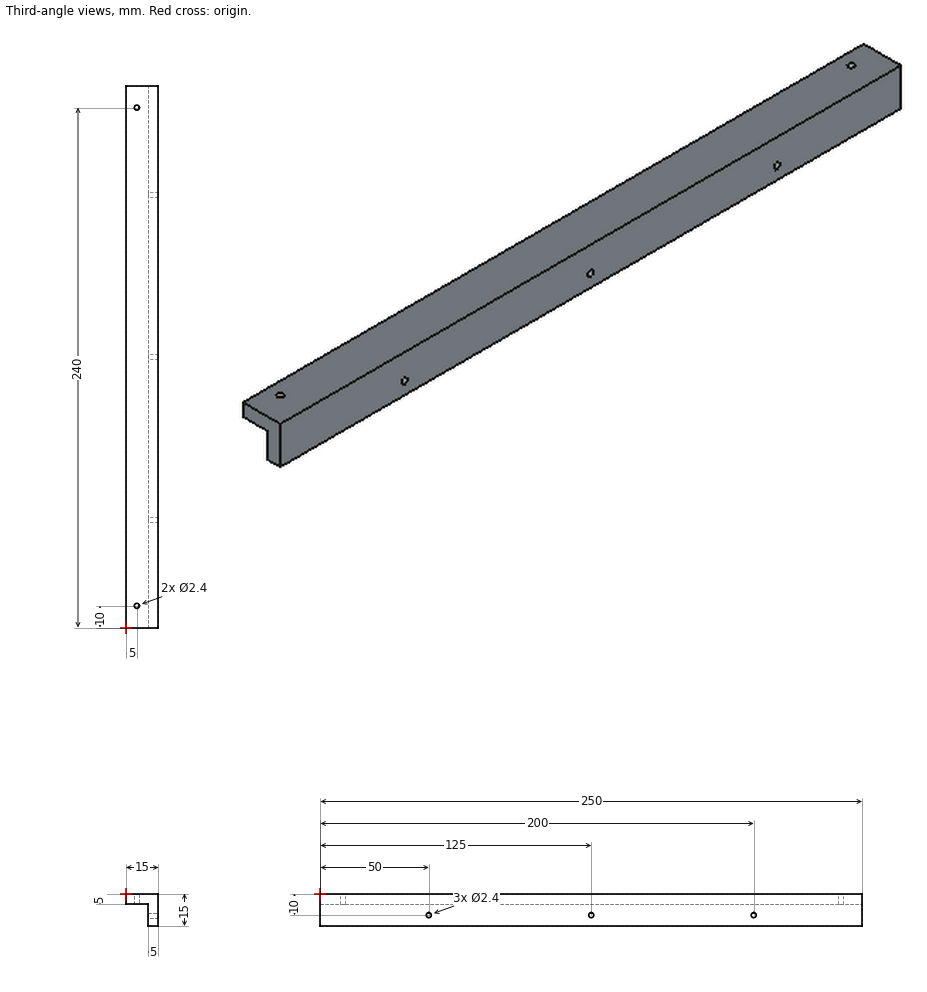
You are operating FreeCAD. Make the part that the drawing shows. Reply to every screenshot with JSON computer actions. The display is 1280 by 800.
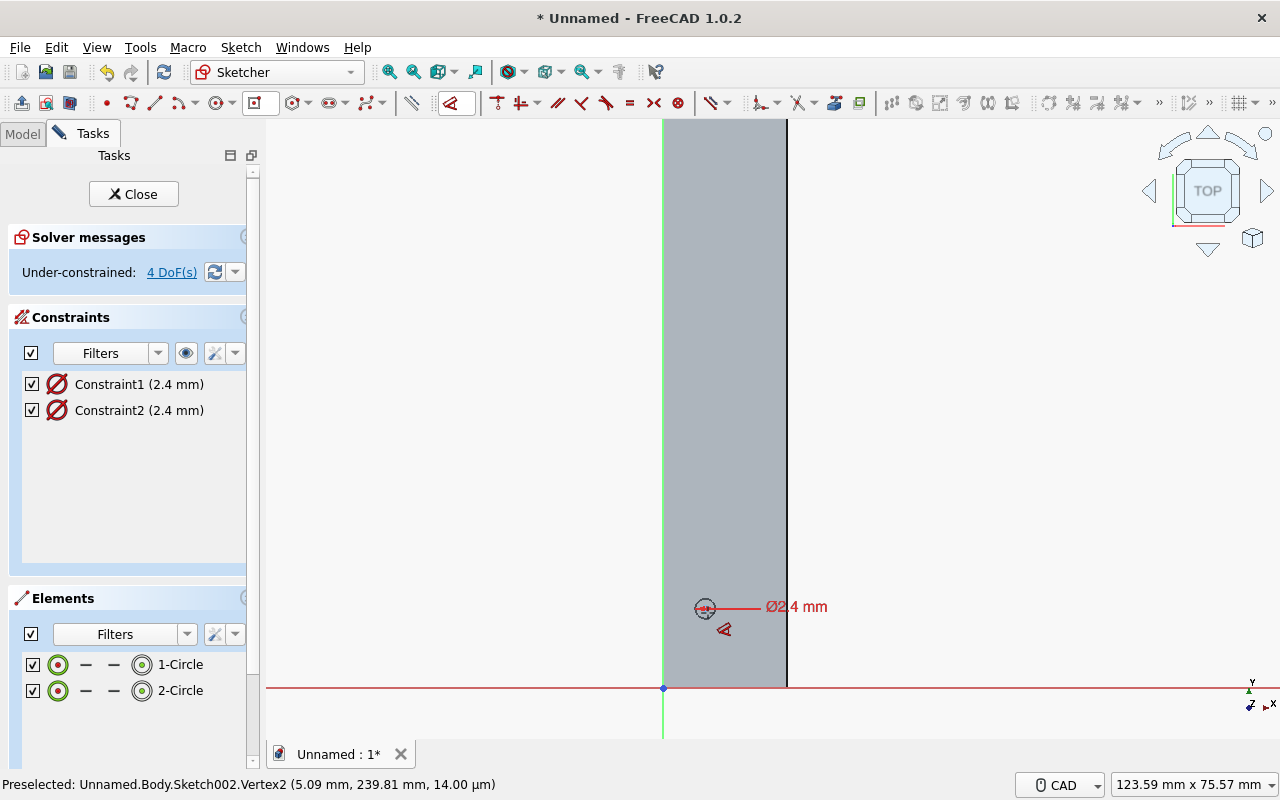
{"action": "left_click", "coordinate": [705, 609]}
{"action": "left_click", "coordinate": [684, 575]}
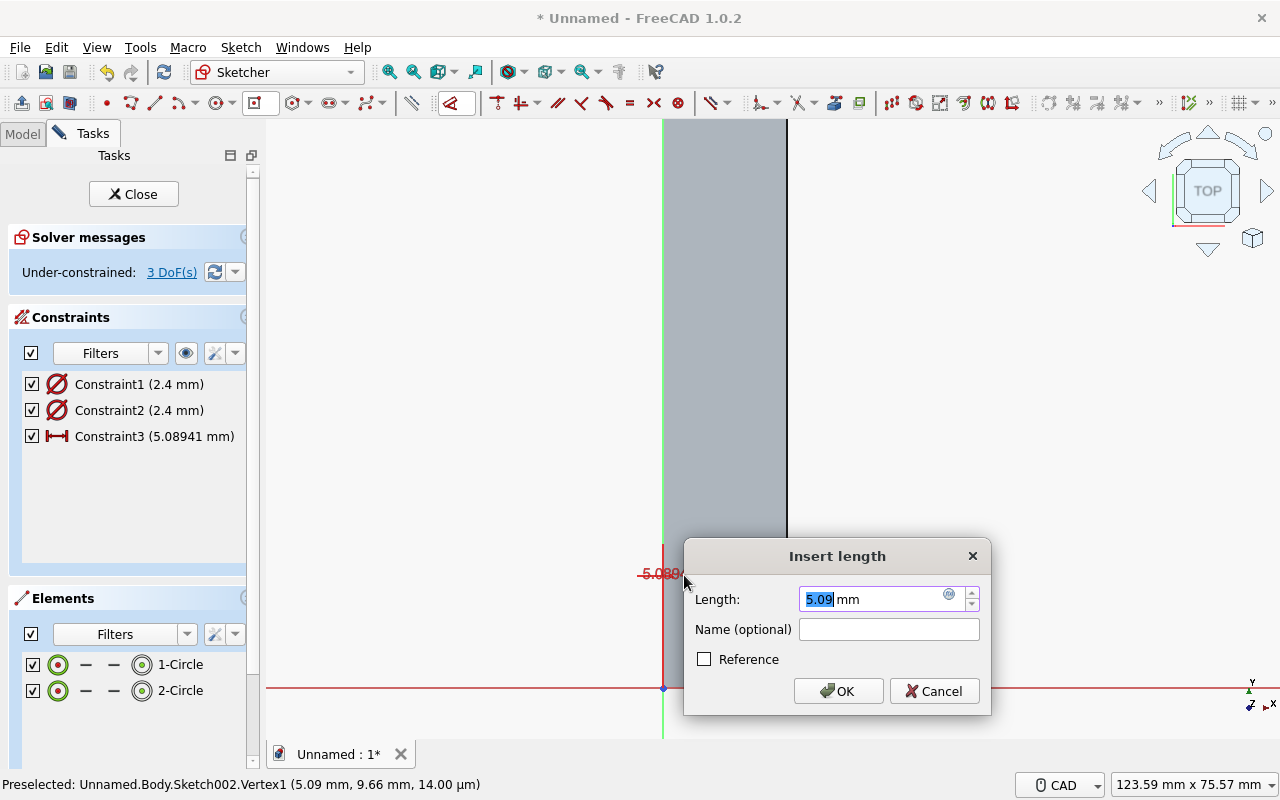
{"action": "type", "text": "5"}
{"action": "key", "text": "Return"}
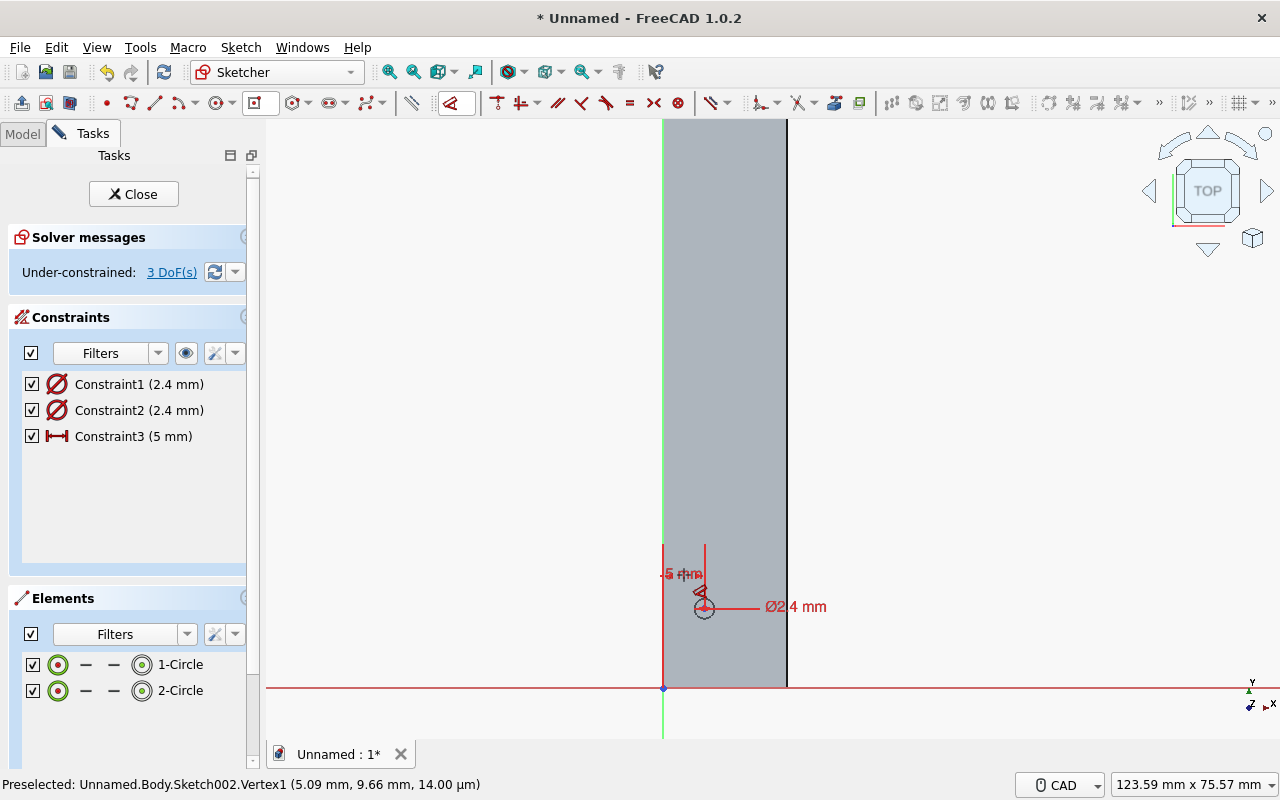
{"action": "scroll", "coordinate": [708, 614], "scroll_direction": "down", "scroll_amount": 8}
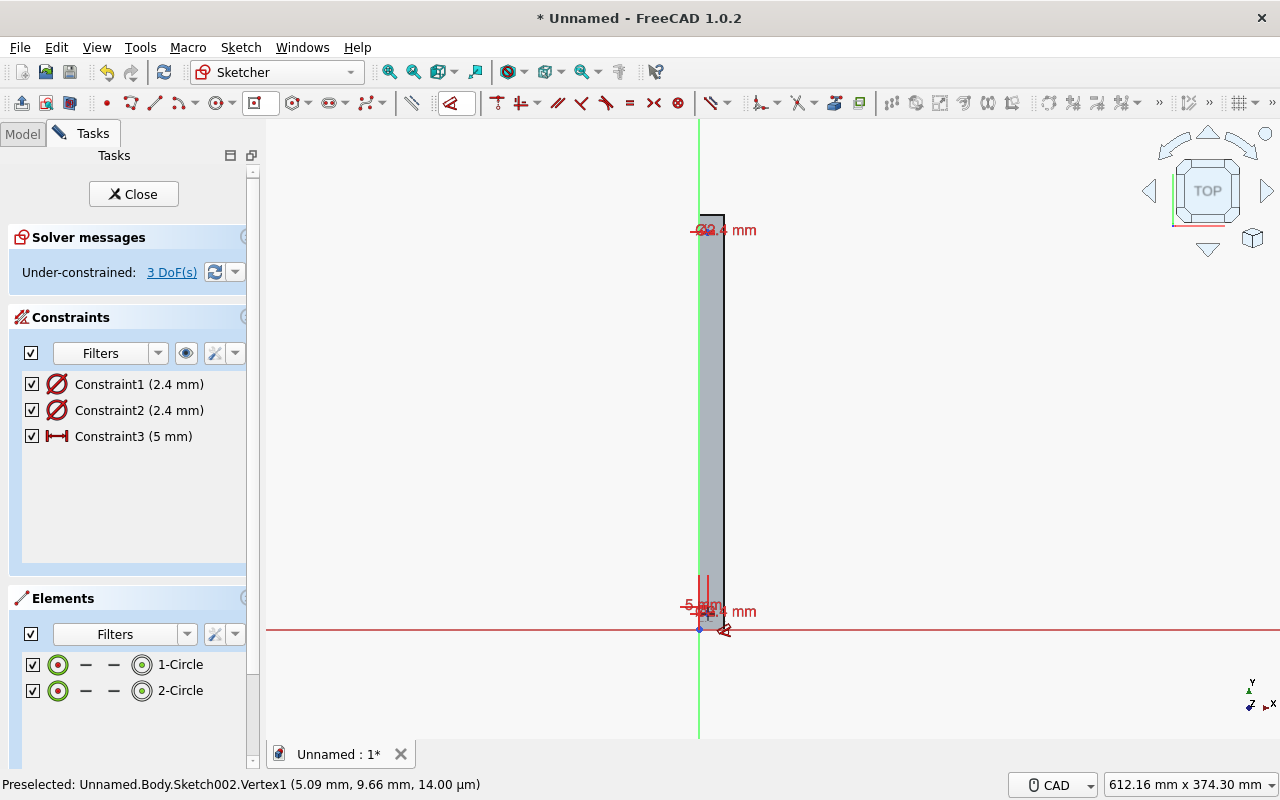
{"action": "scroll", "coordinate": [708, 232], "scroll_direction": "up", "scroll_amount": 8}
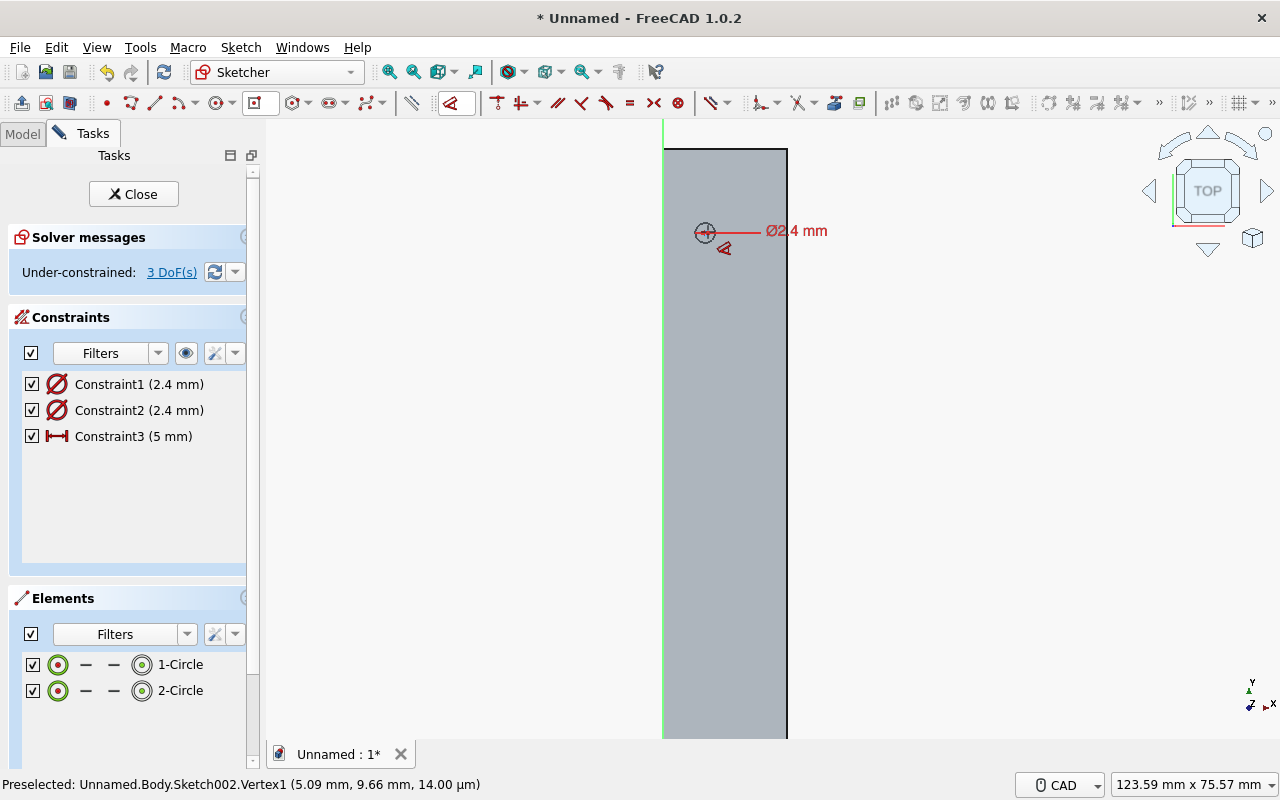
{"action": "left_click", "coordinate": [705, 233]}
{"action": "left_click", "coordinate": [684, 199]}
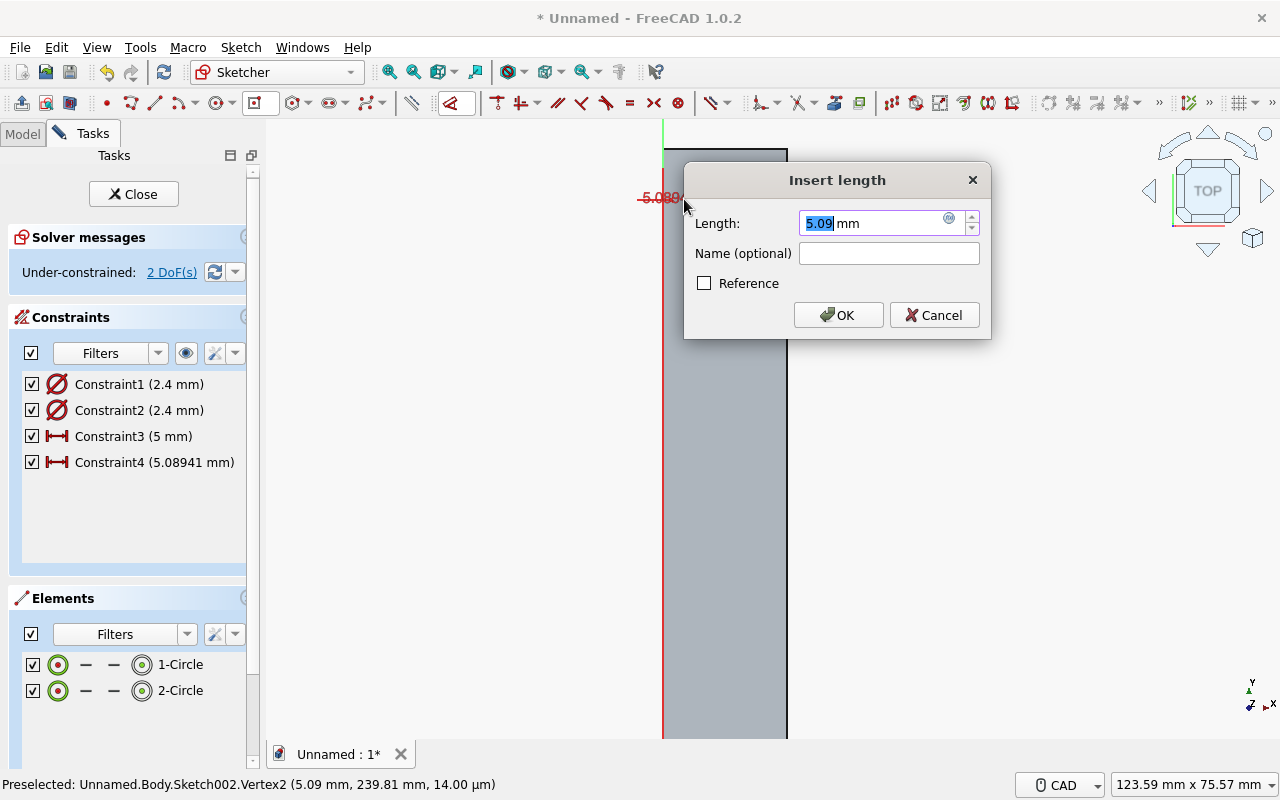
{"action": "type", "text": "5"}
{"action": "key", "text": "Return"}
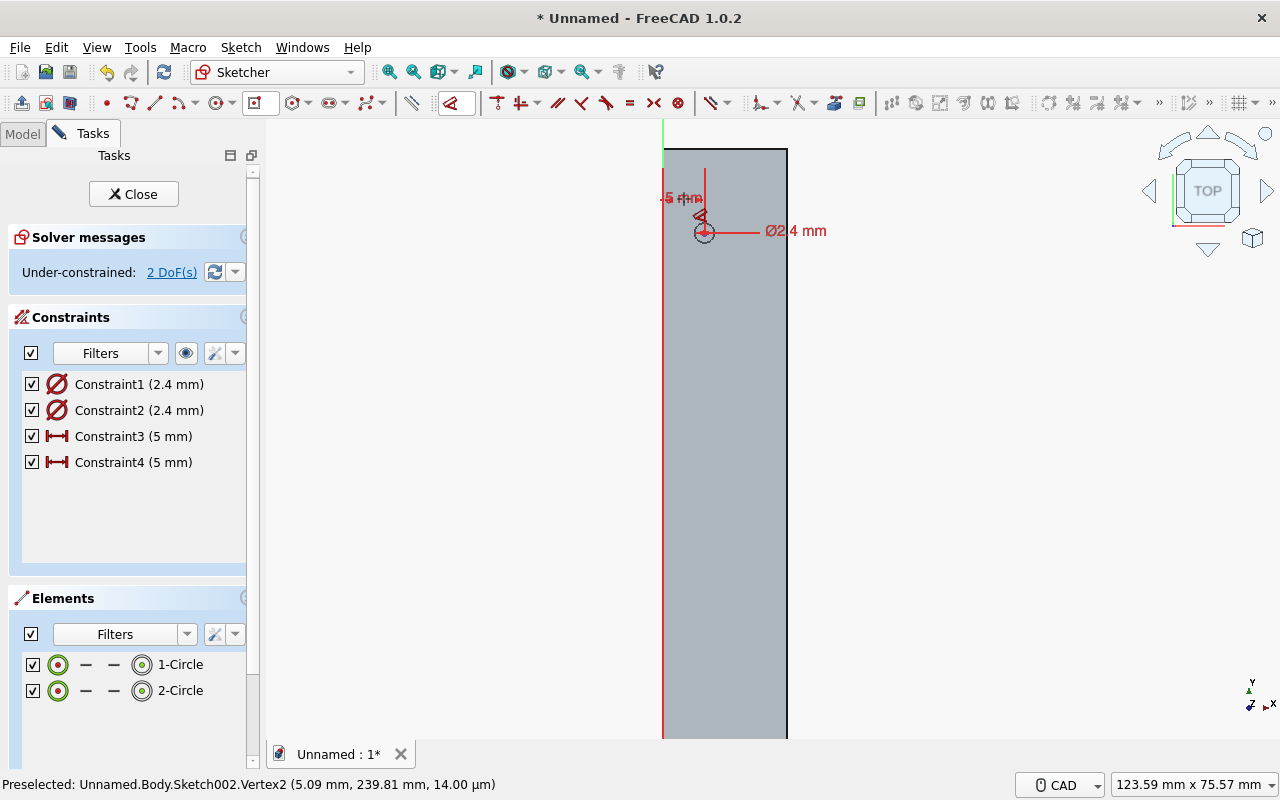
{"action": "scroll", "coordinate": [708, 231], "scroll_direction": "down", "scroll_amount": 8}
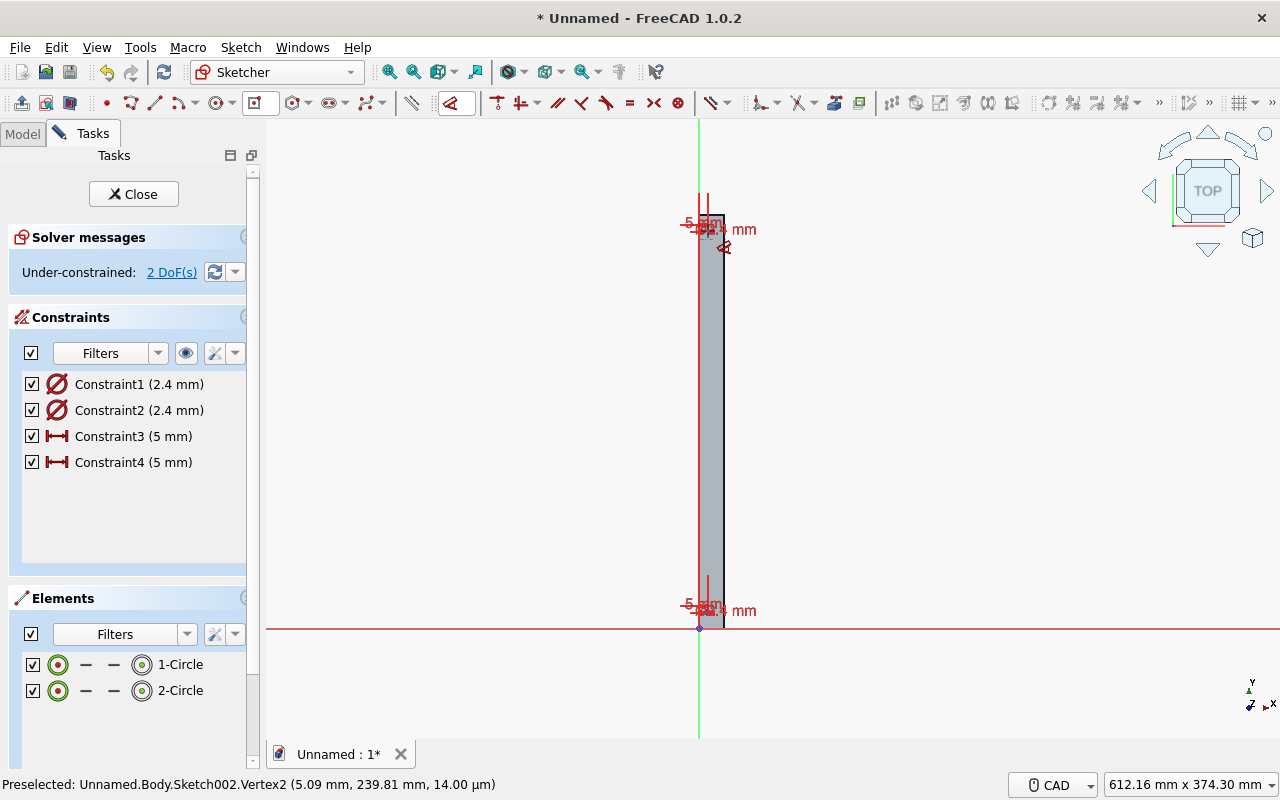
{"action": "scroll", "coordinate": [708, 613], "scroll_direction": "up", "scroll_amount": 5}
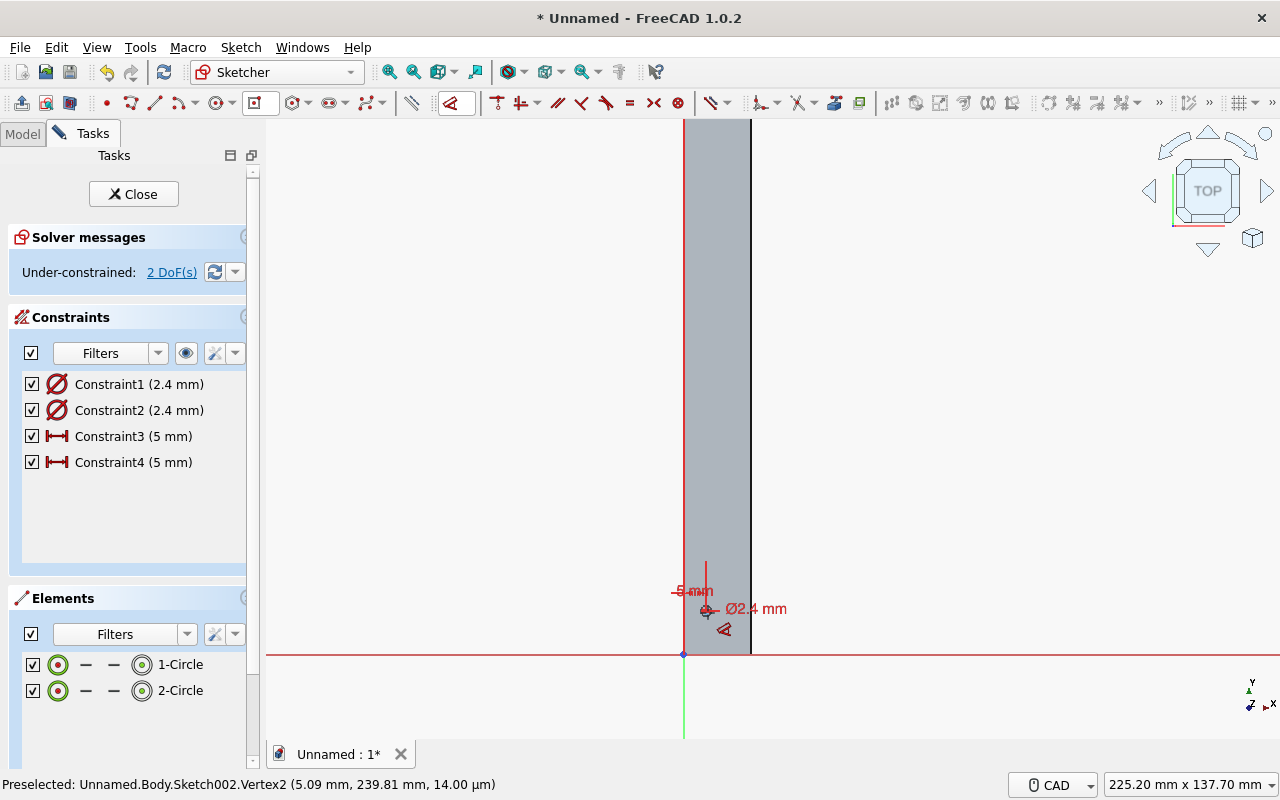
{"action": "left_click", "coordinate": [706, 611]}
{"action": "left_click", "coordinate": [650, 633]}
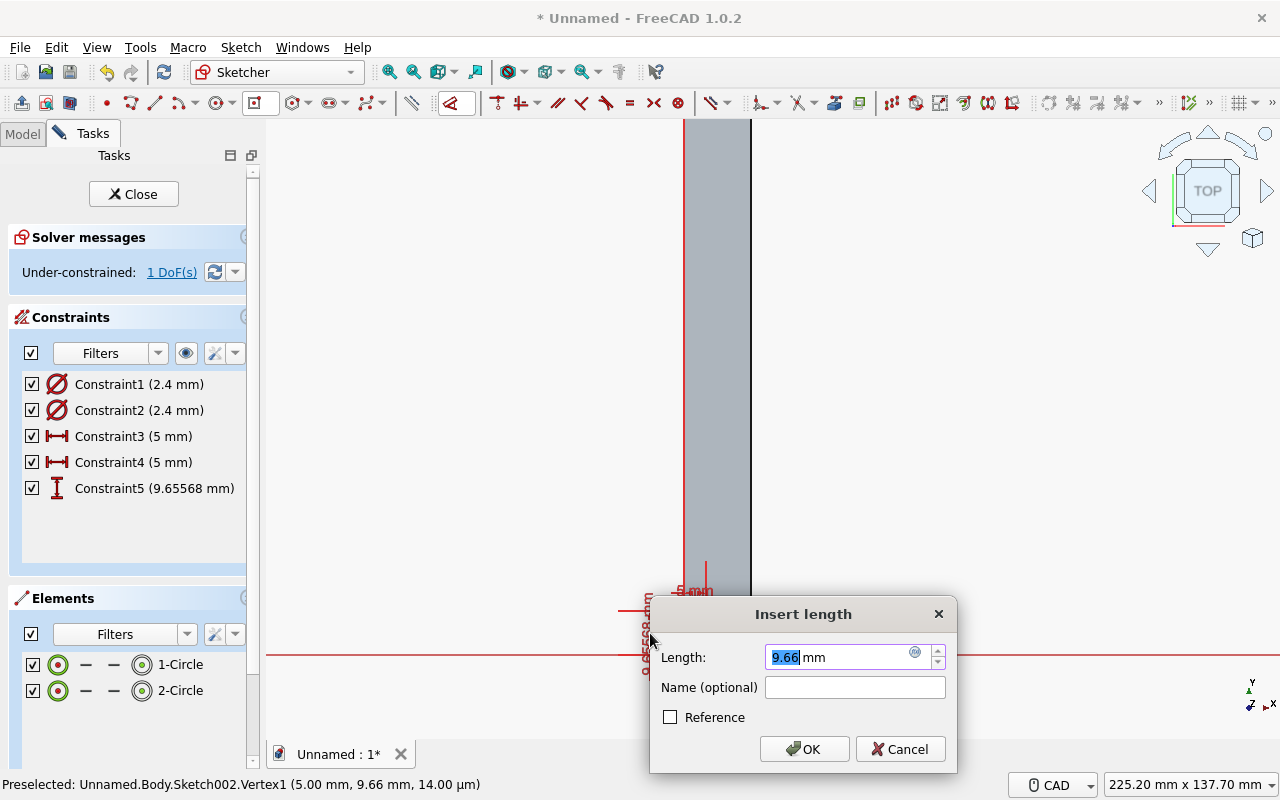
{"action": "type", "text": "10"}
{"action": "key", "text": "Return"}